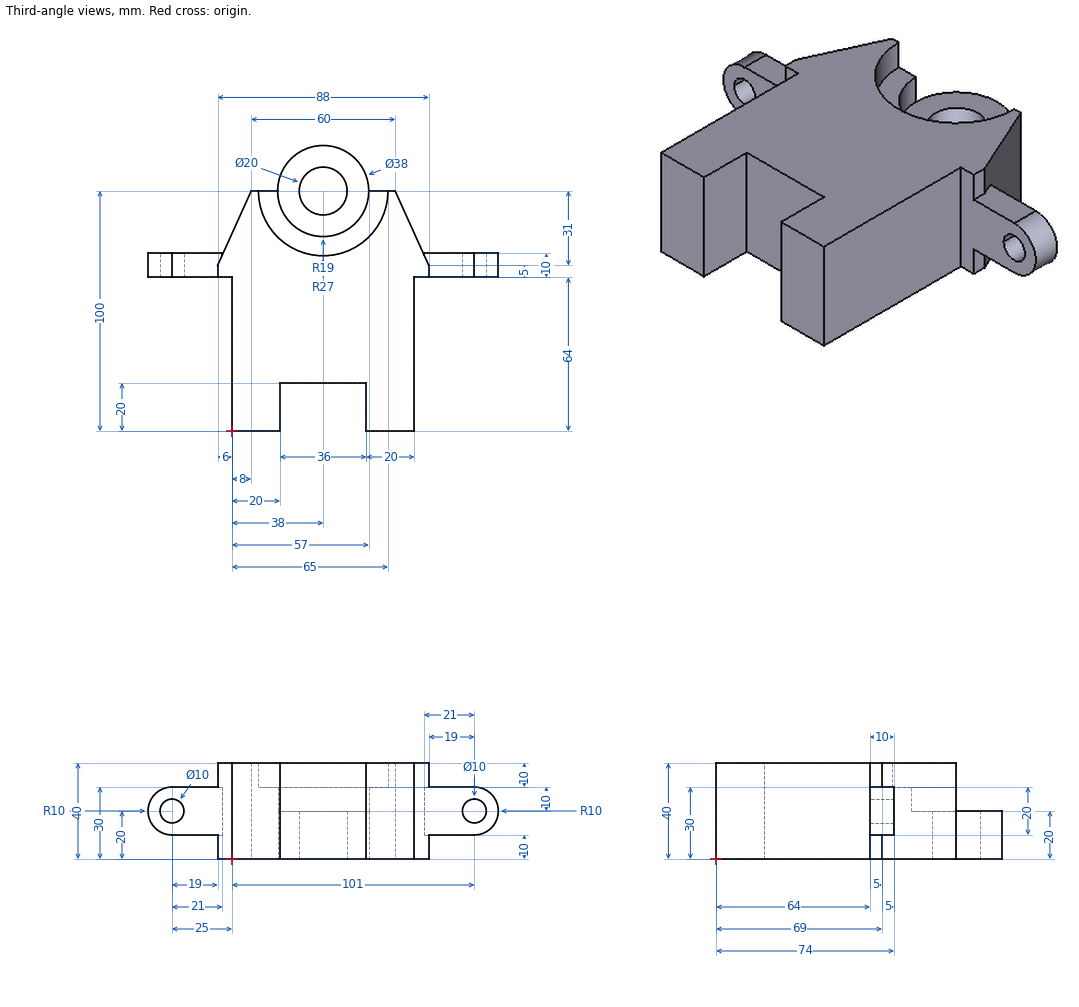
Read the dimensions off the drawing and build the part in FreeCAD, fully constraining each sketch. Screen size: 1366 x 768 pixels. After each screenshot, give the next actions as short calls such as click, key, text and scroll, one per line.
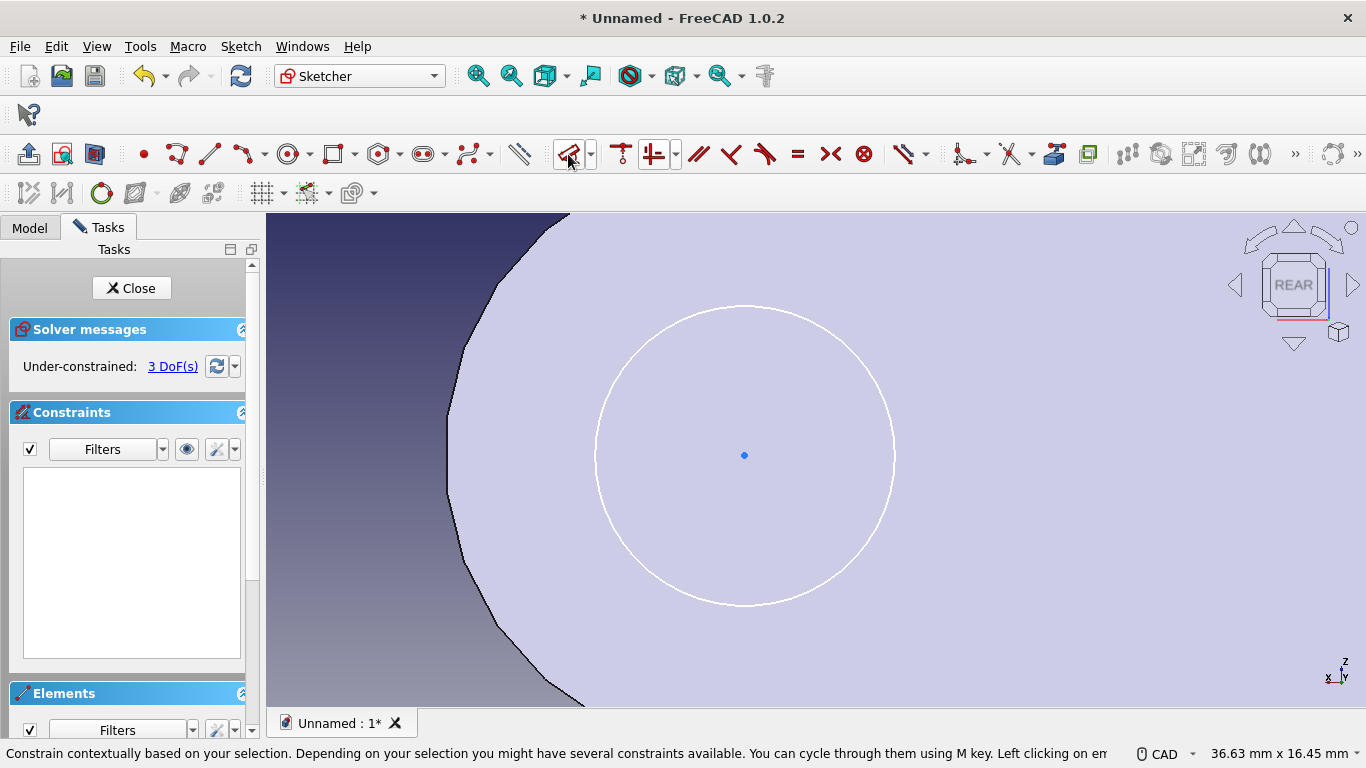
click(851, 350)
click(874, 327)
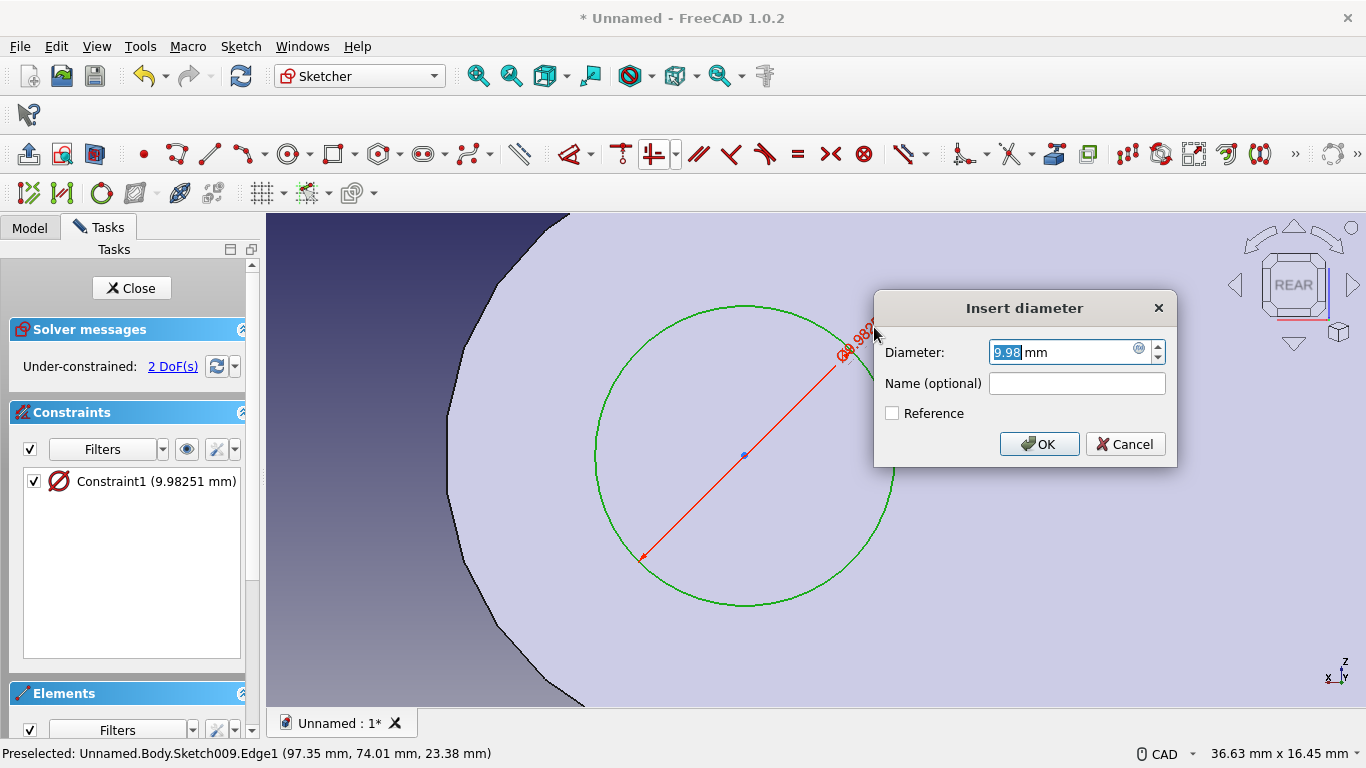
text(10)
key(Return)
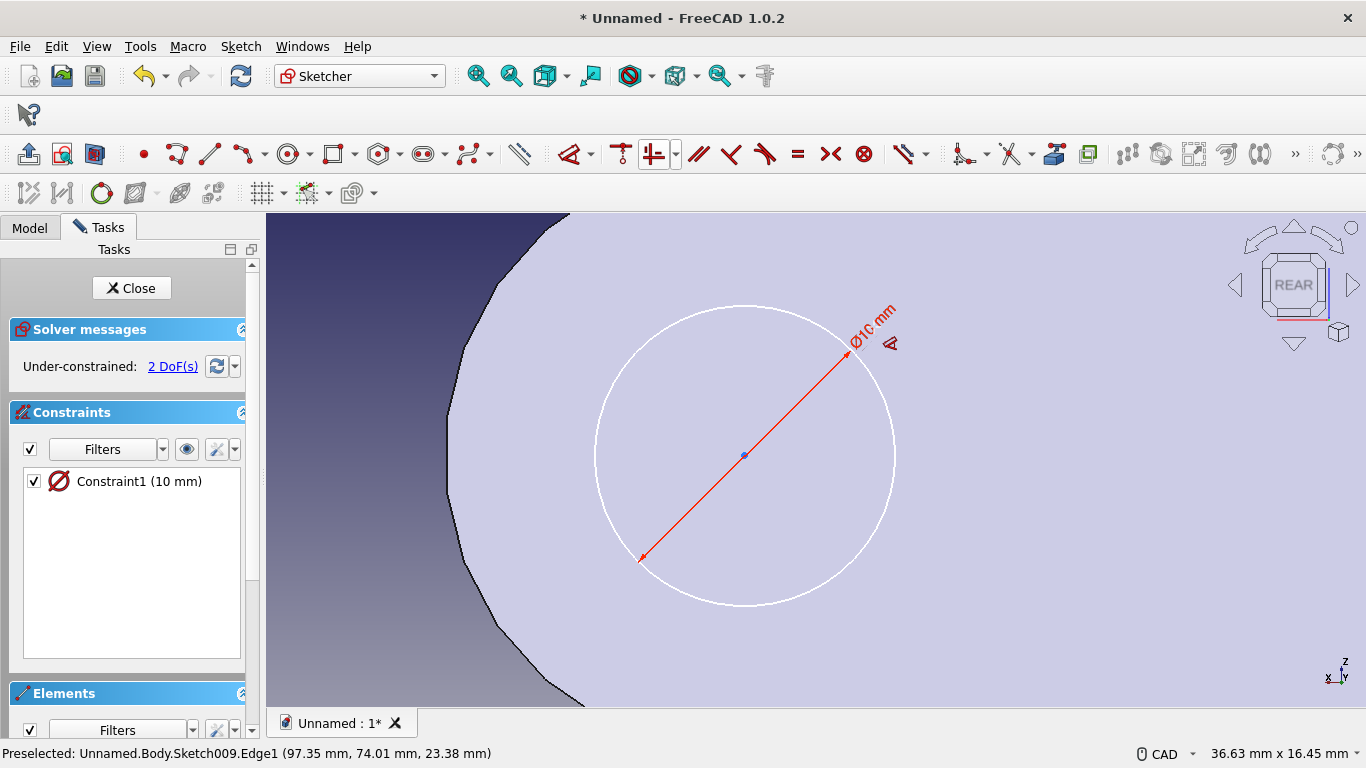
click(745, 456)
click(711, 568)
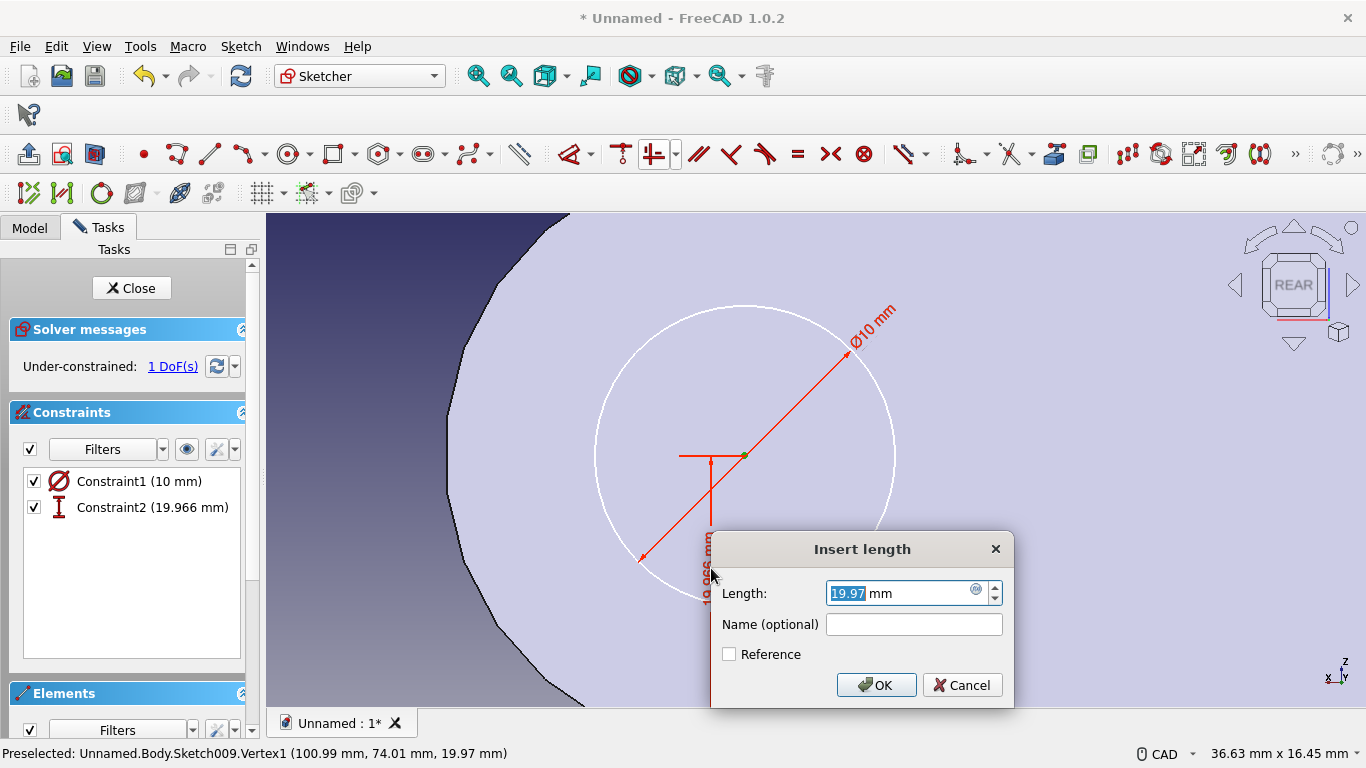
text(20)
key(Return)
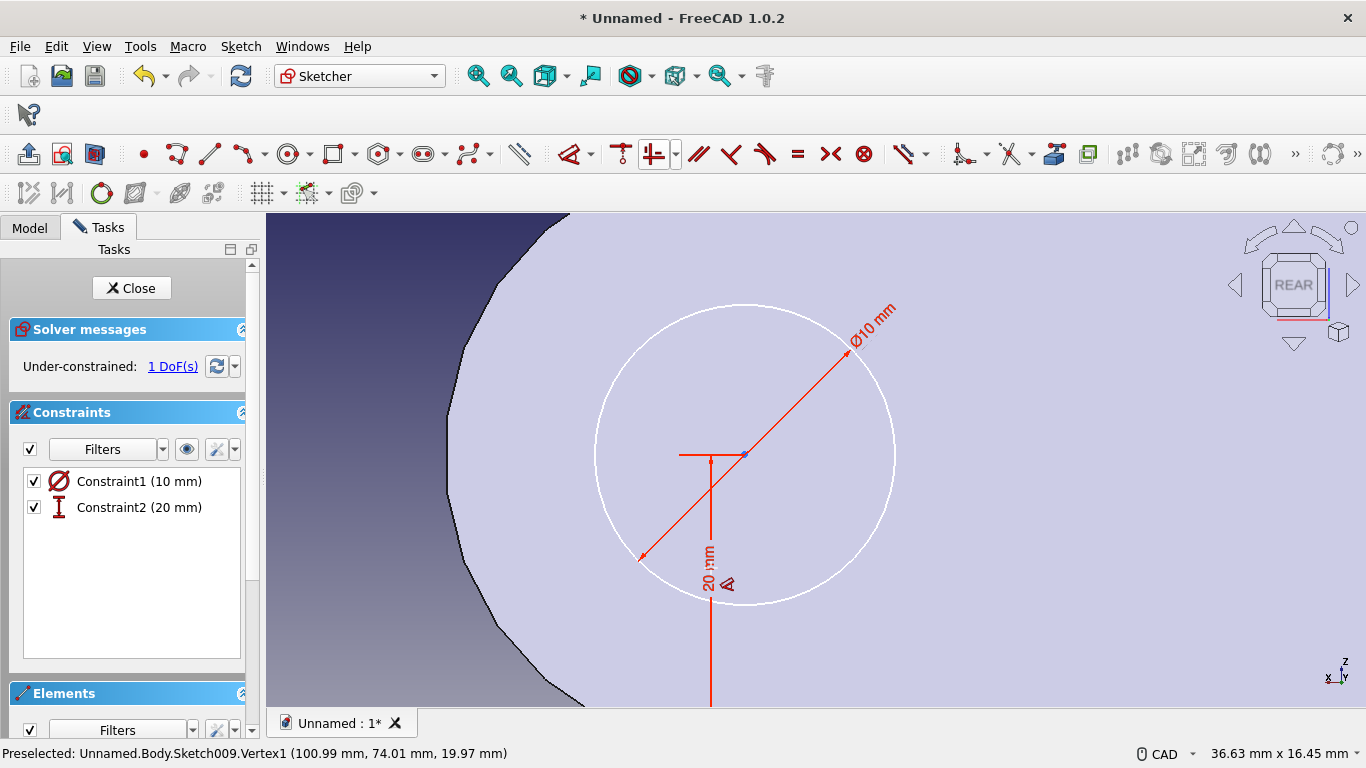
click(745, 455)
click(973, 421)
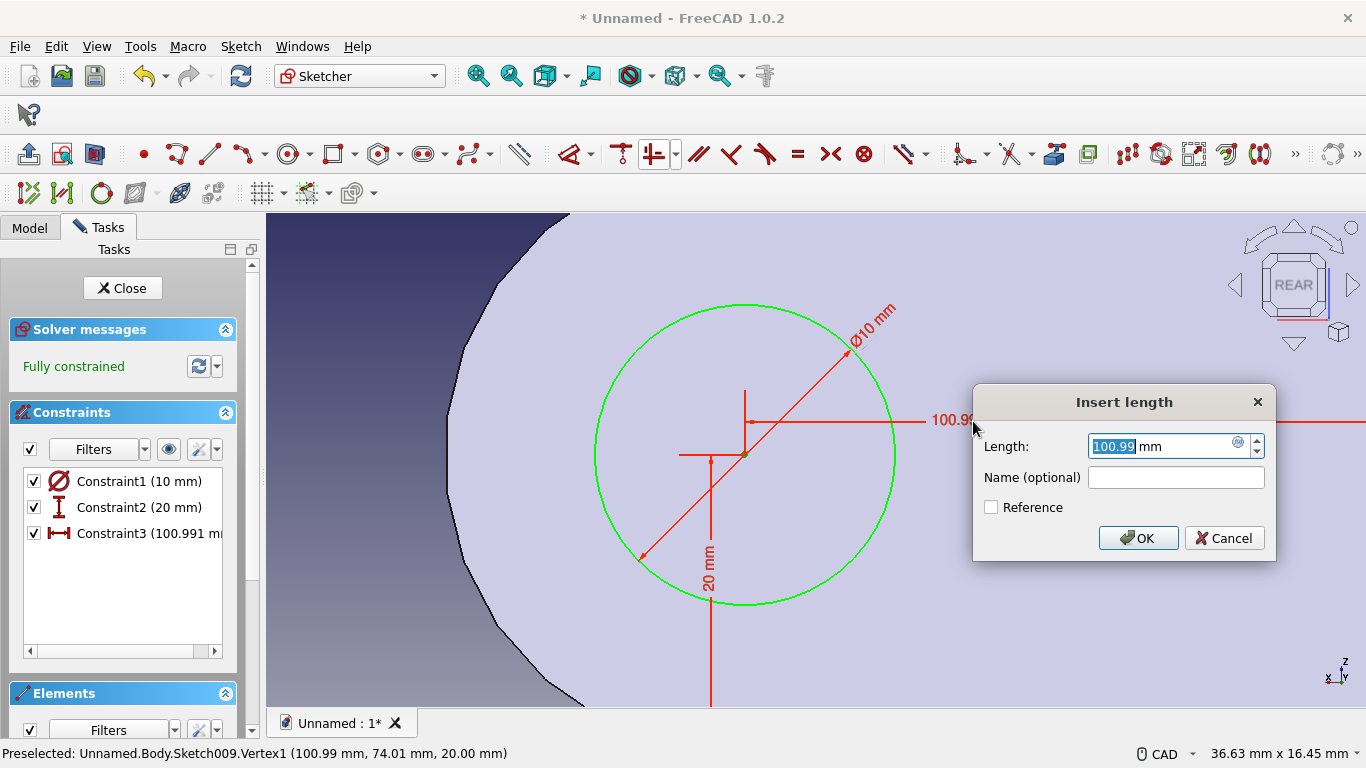
text(101)
key(Return)
key(Escape)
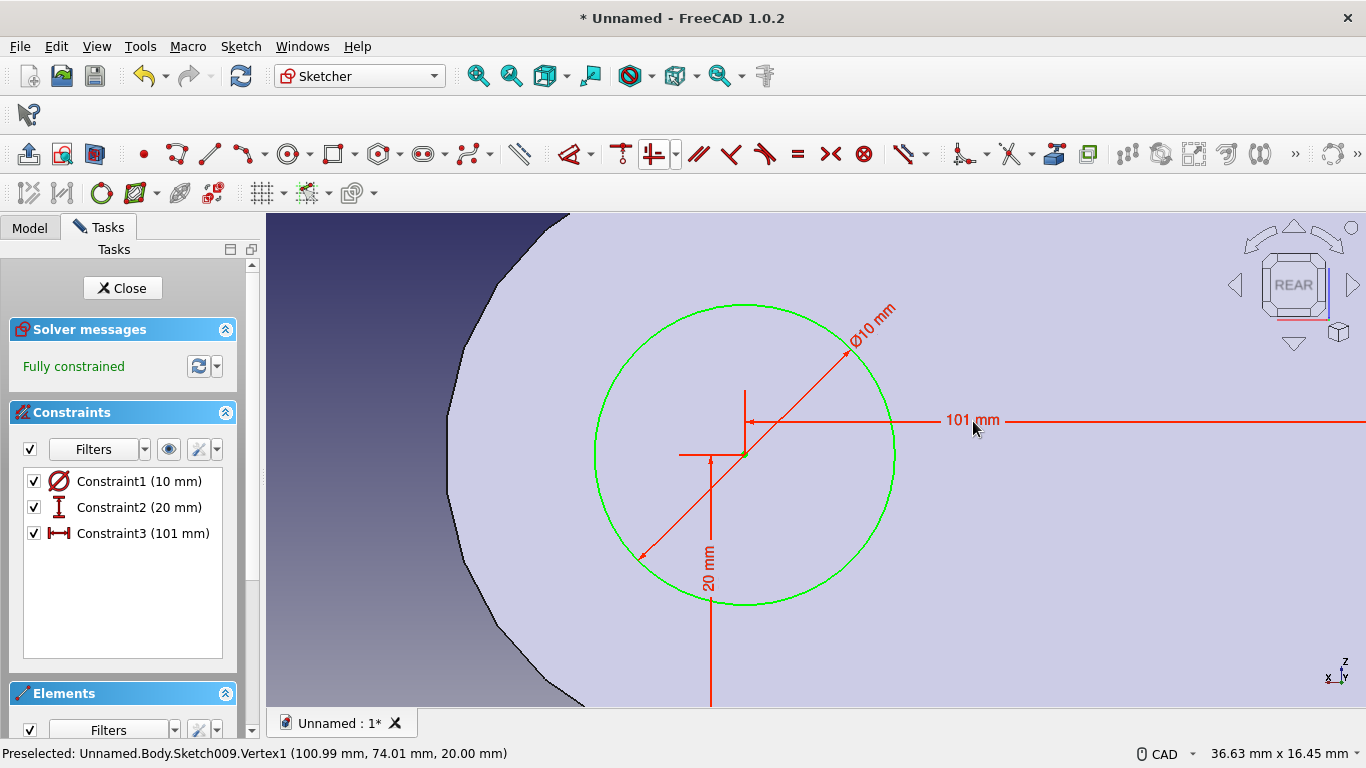
click(123, 288)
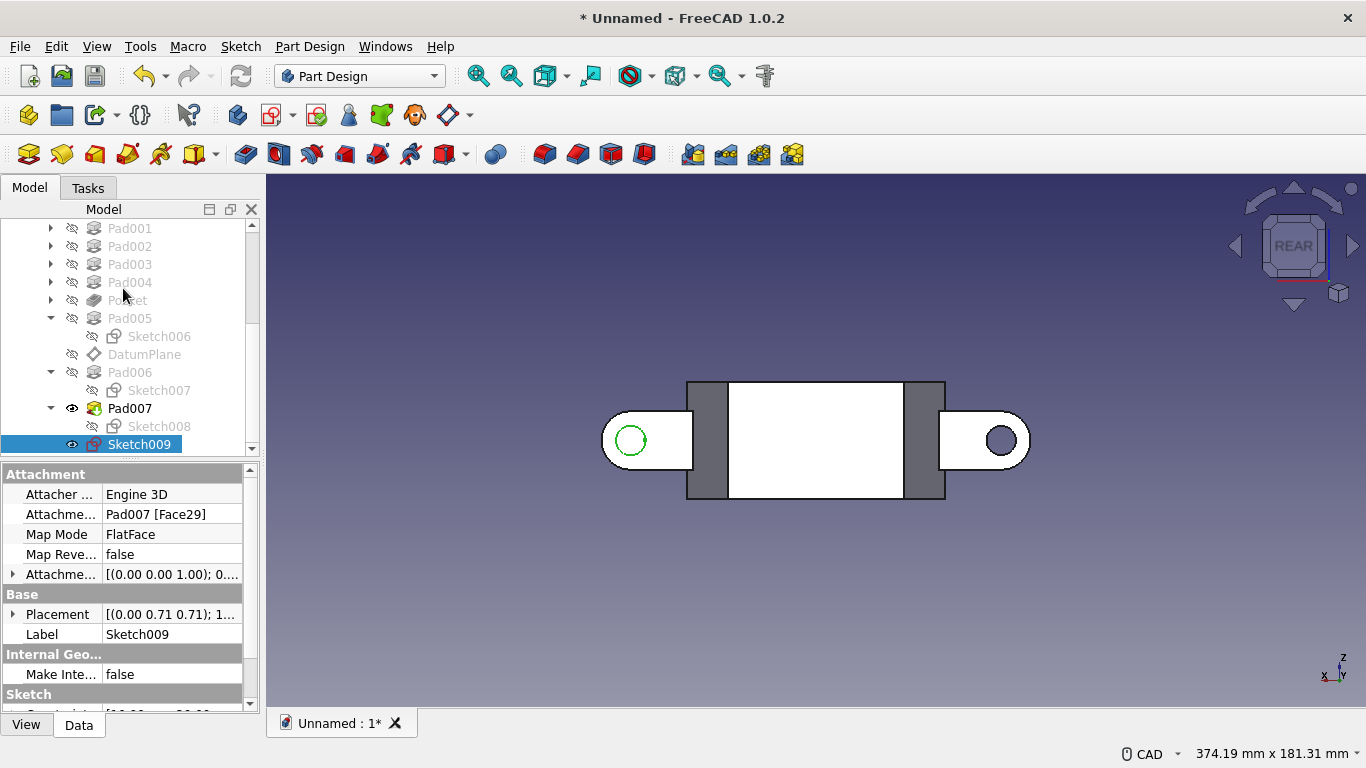
click(246, 154)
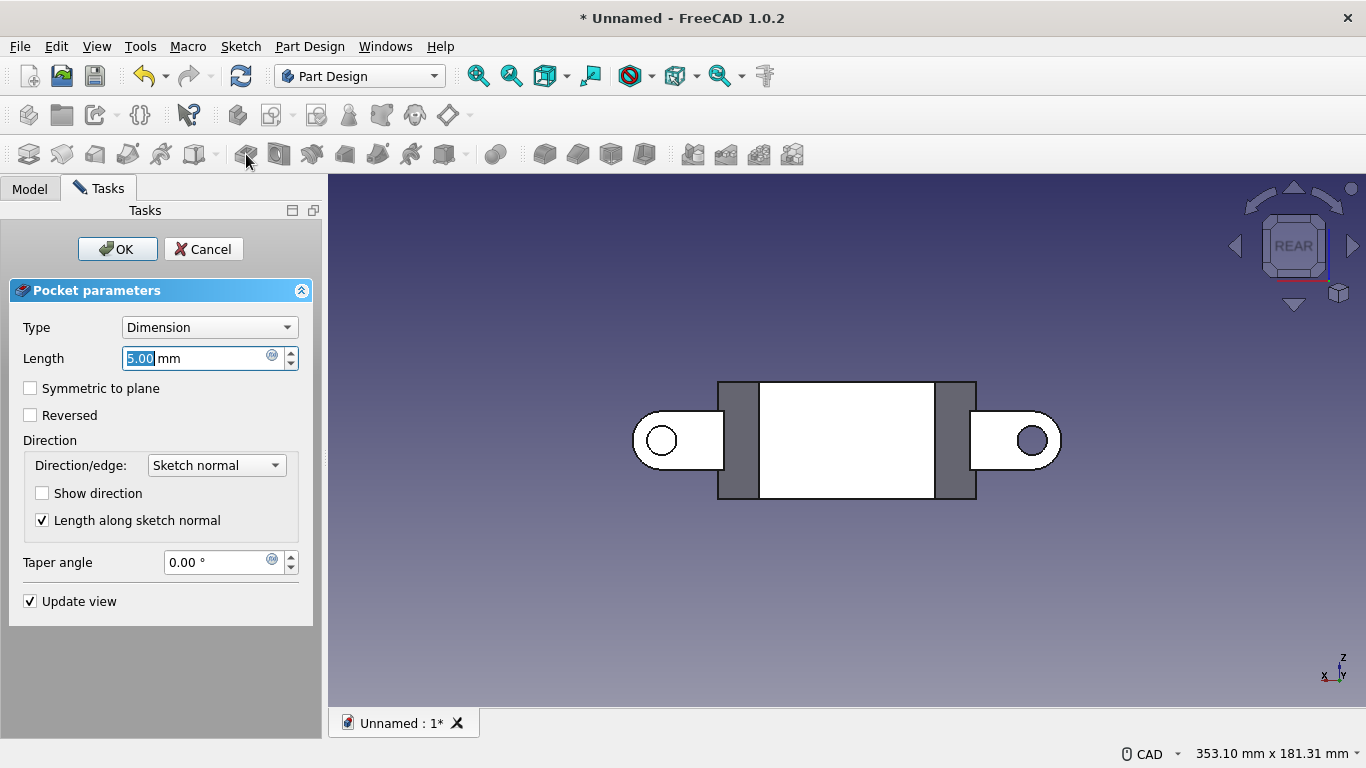
text(10)
key(Tab)